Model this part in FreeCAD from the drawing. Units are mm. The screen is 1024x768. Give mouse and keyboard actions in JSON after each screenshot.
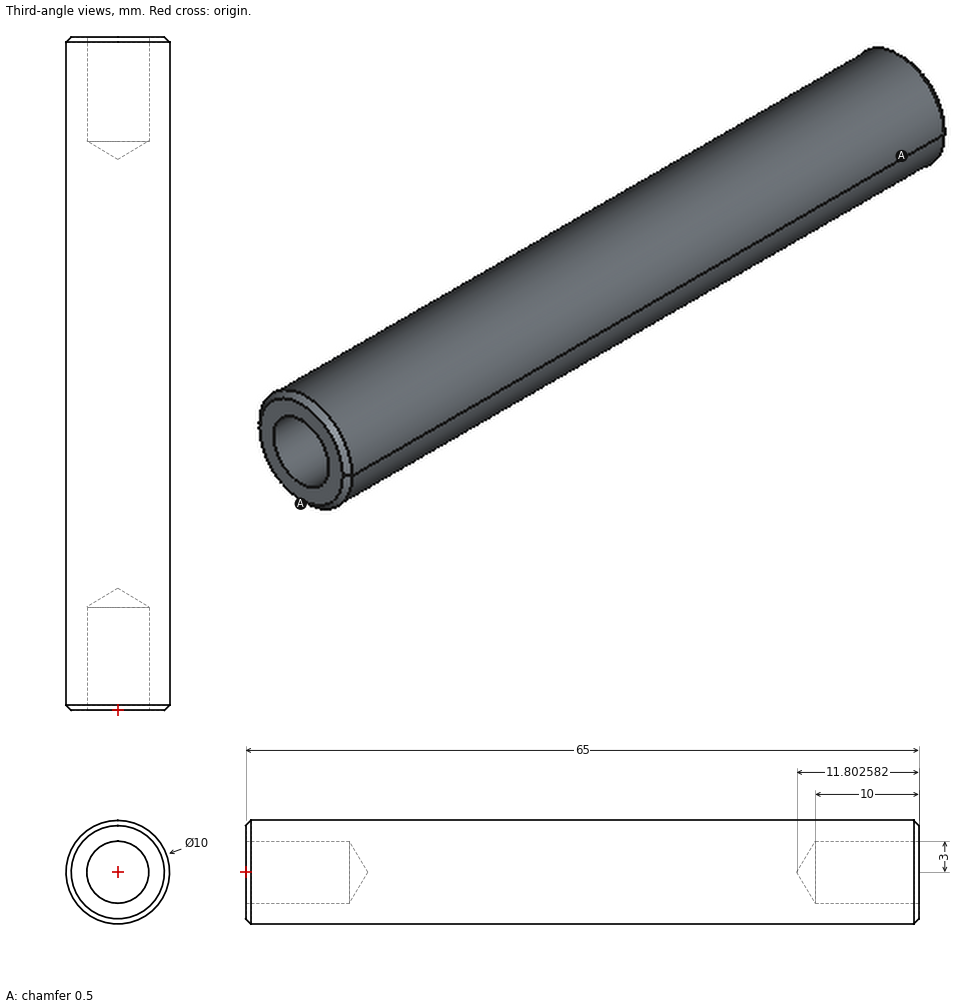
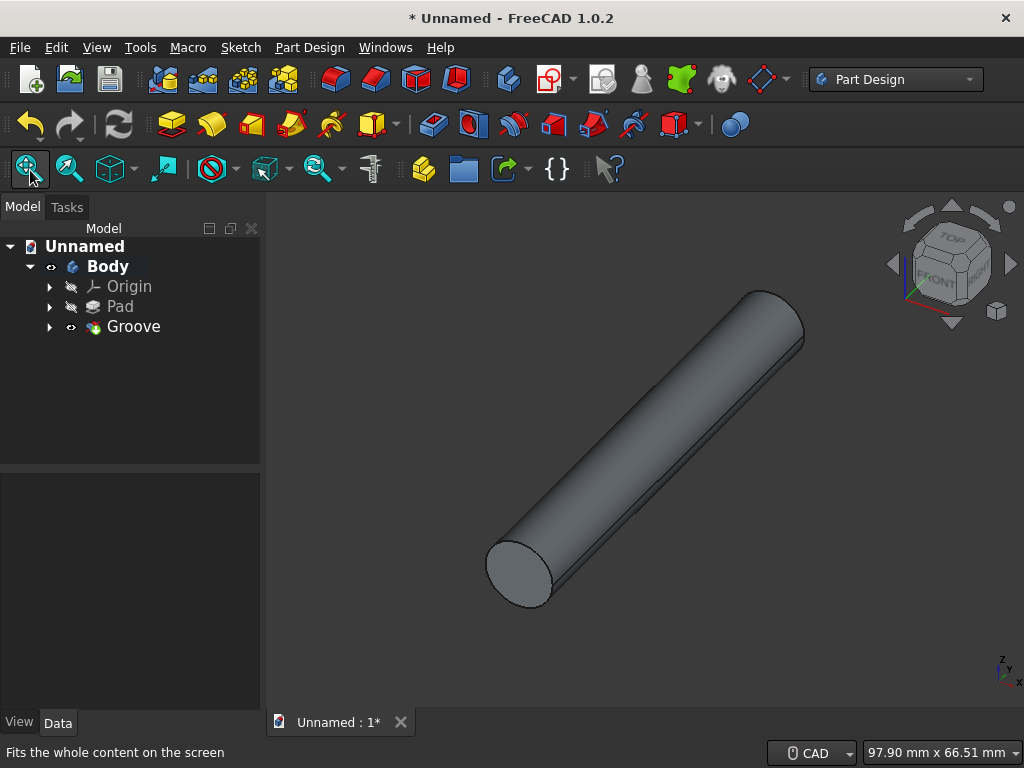
{"action": "left_click", "coordinate": [50, 287]}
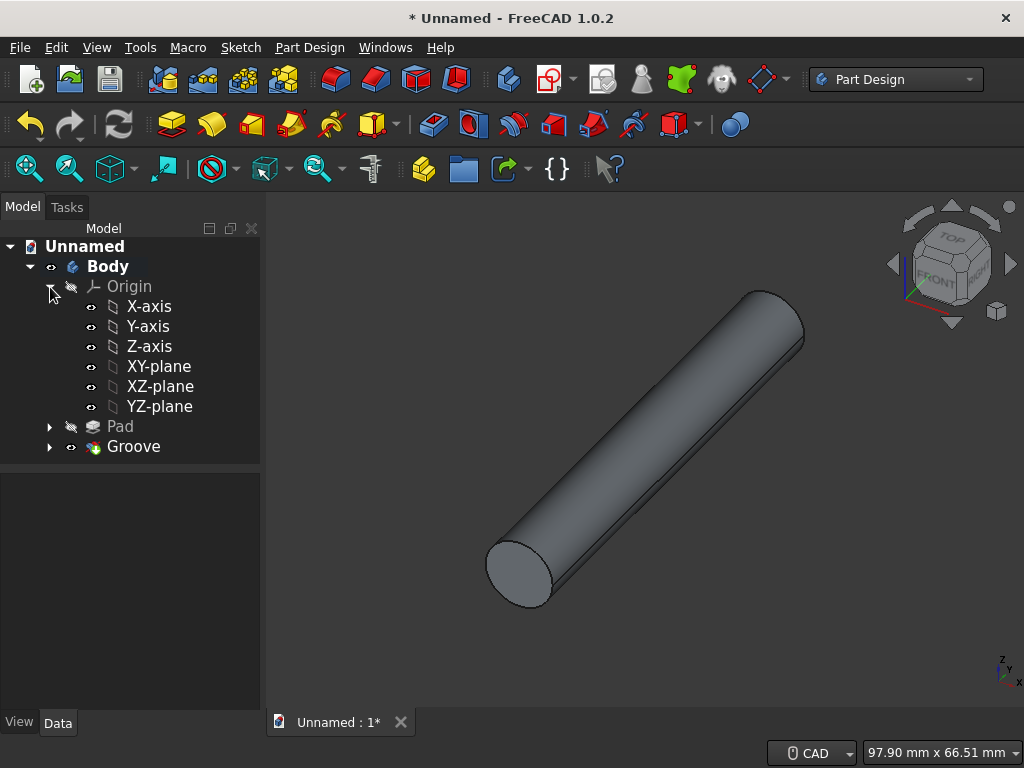
{"action": "left_click", "coordinate": [136, 387]}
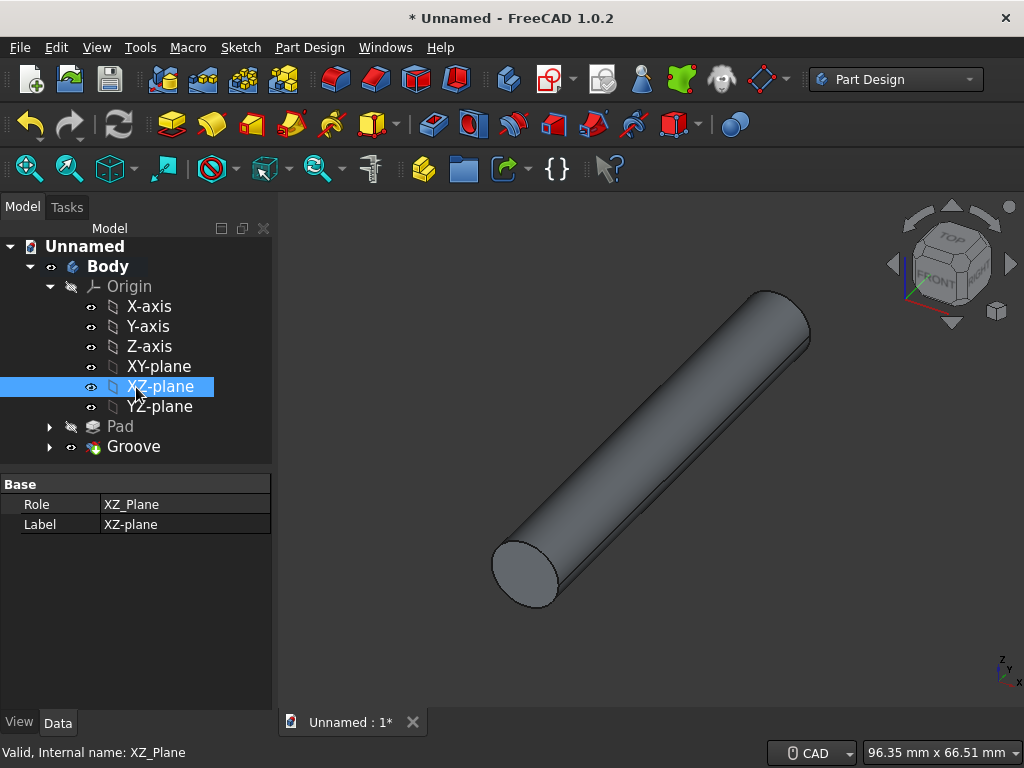
{"action": "left_click", "coordinate": [762, 80]}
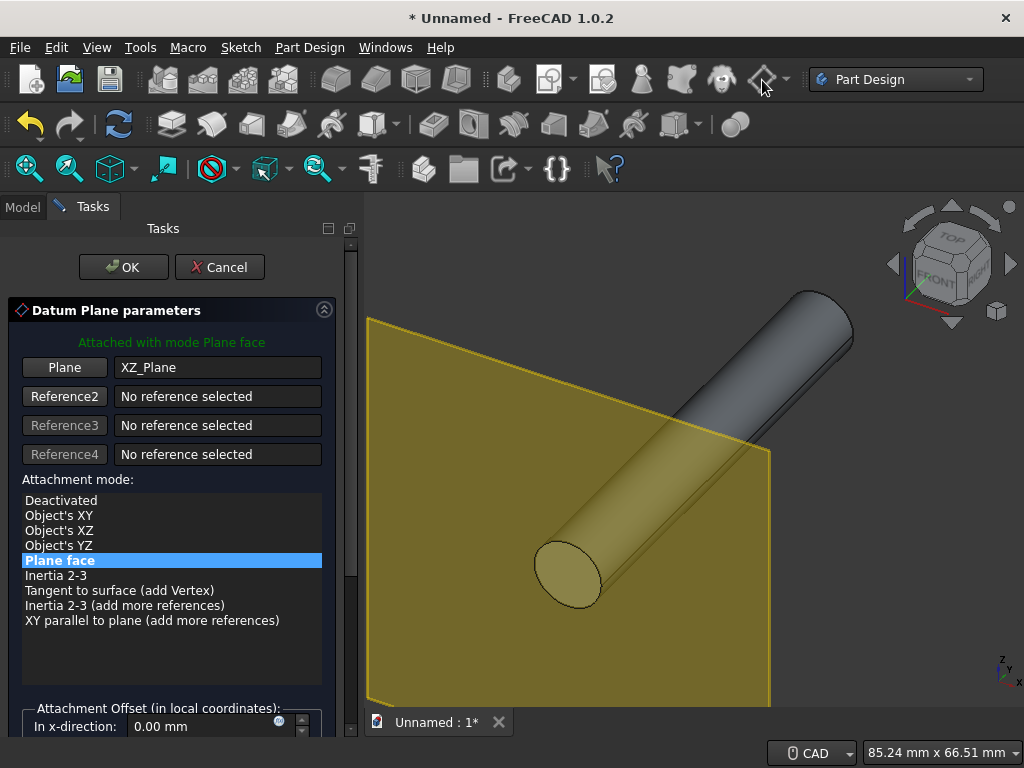
{"action": "scroll", "coordinate": [351, 487], "scroll_direction": "down", "scroll_amount": 3}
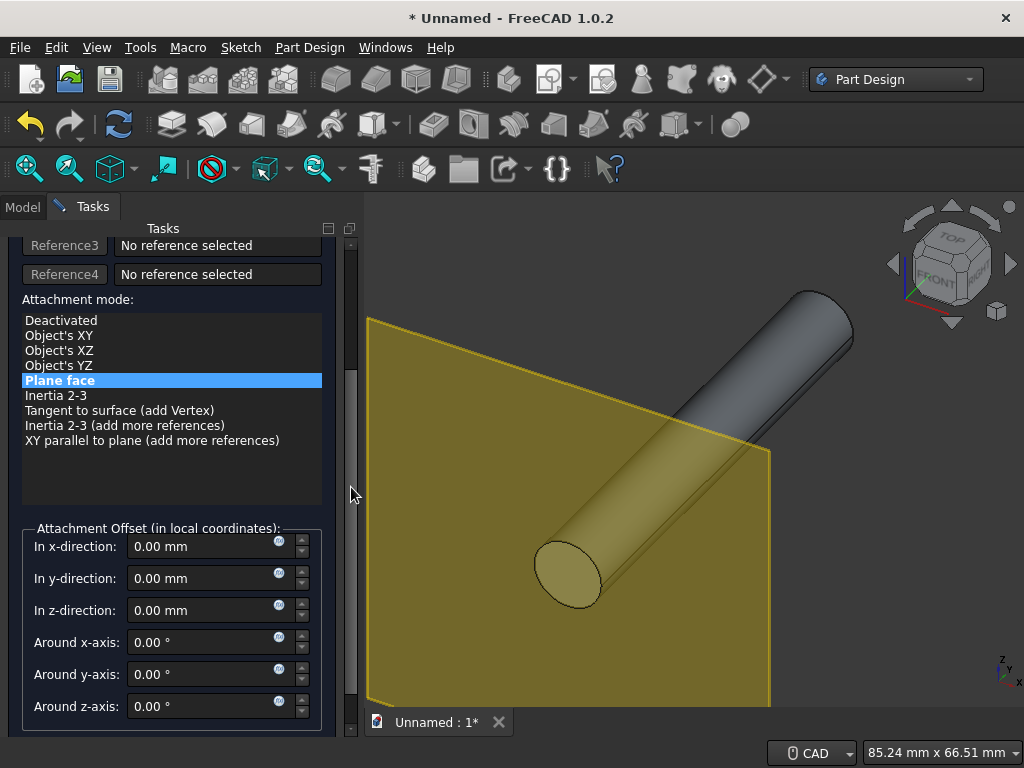
{"action": "triple_click", "coordinate": [210, 610]}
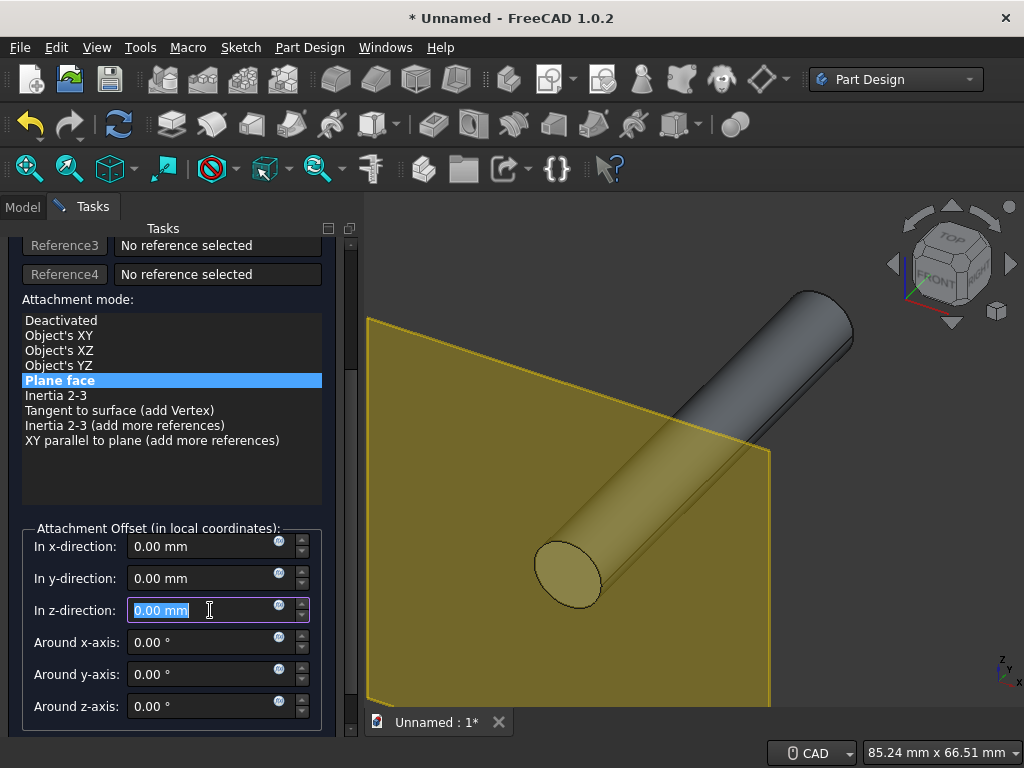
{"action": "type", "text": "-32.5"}
{"action": "key", "text": "Tab"}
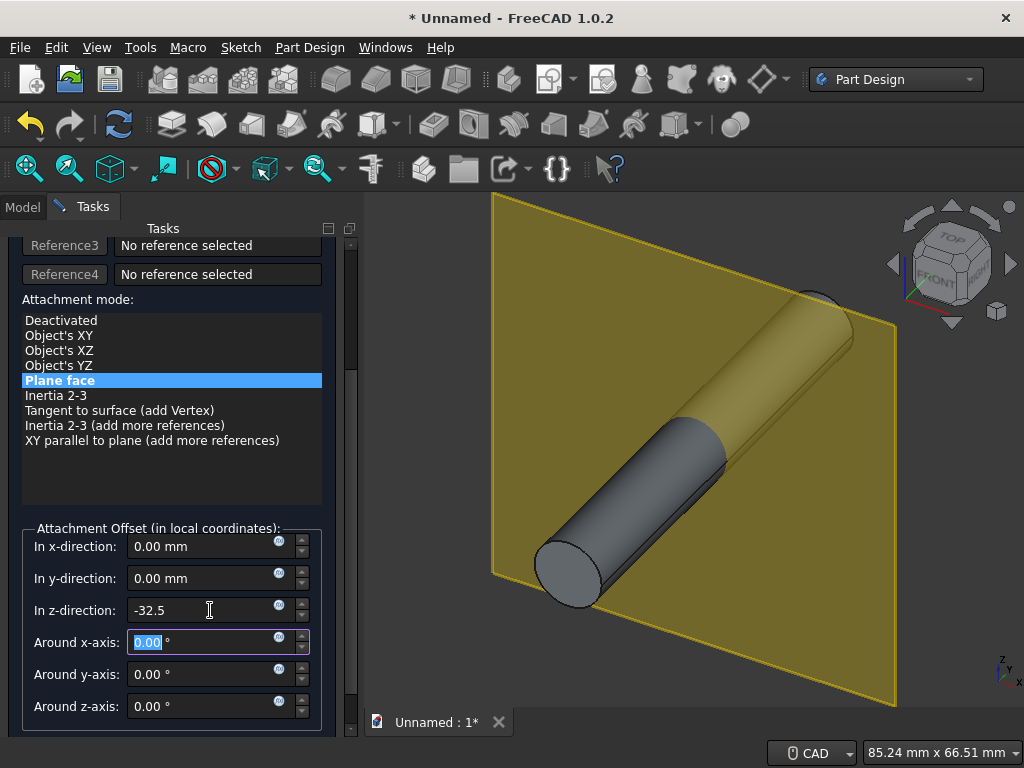
{"action": "scroll", "coordinate": [351, 487], "scroll_direction": "up", "scroll_amount": 4}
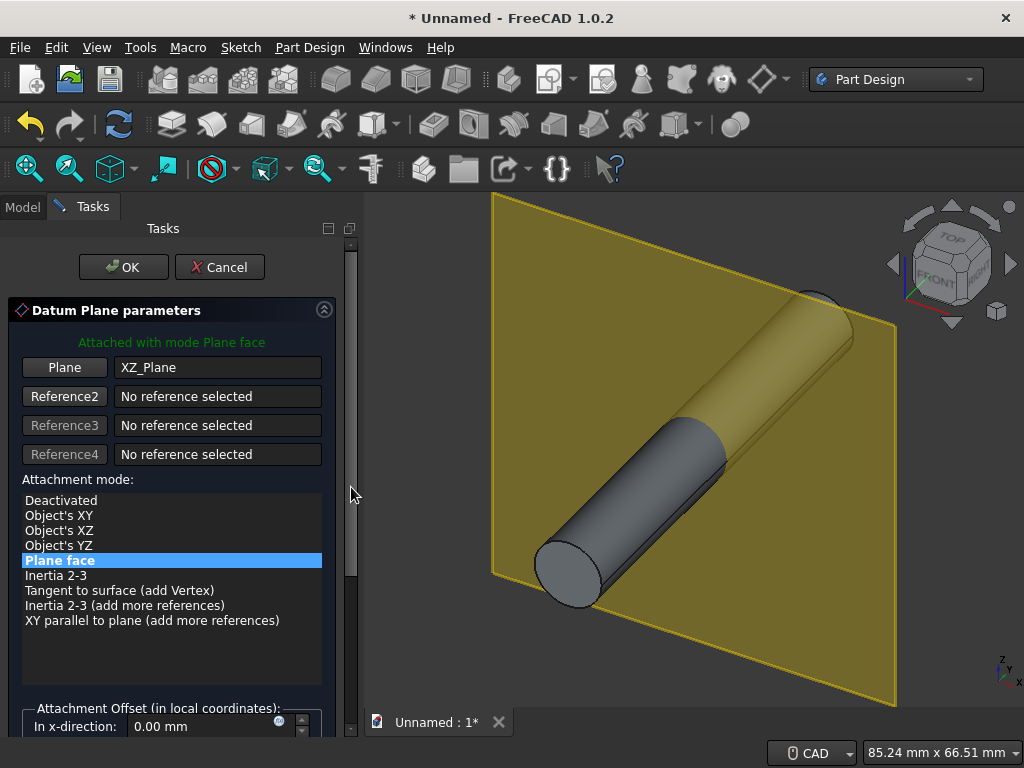
{"action": "left_click", "coordinate": [124, 267]}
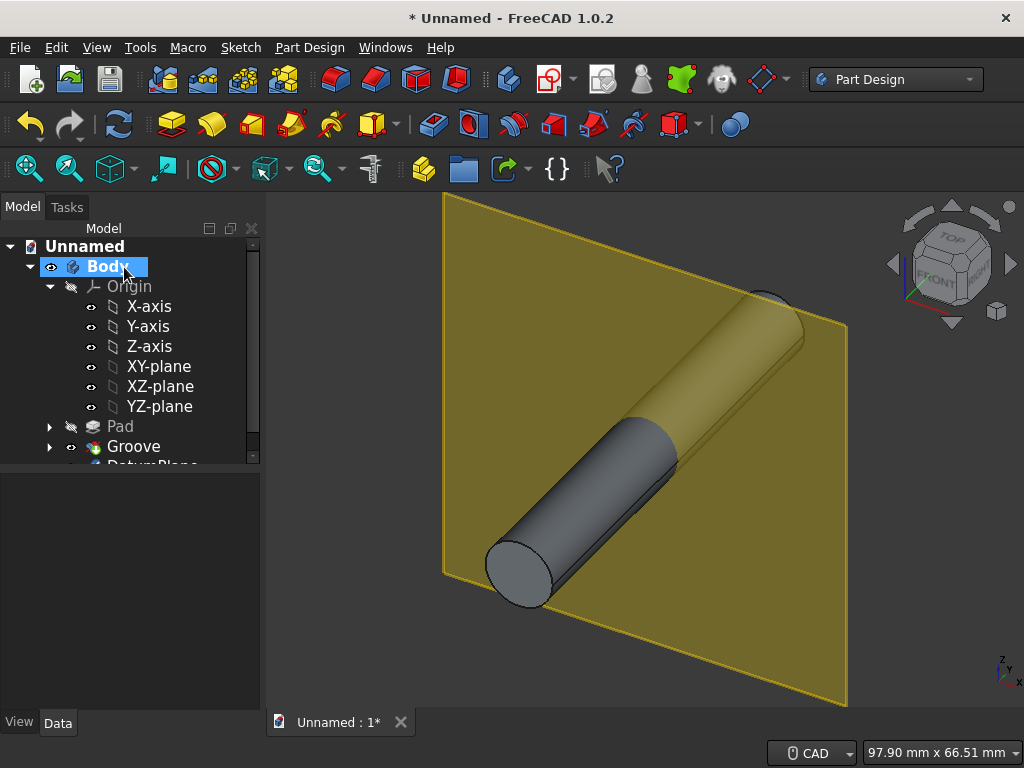
{"action": "left_click", "coordinate": [116, 447]}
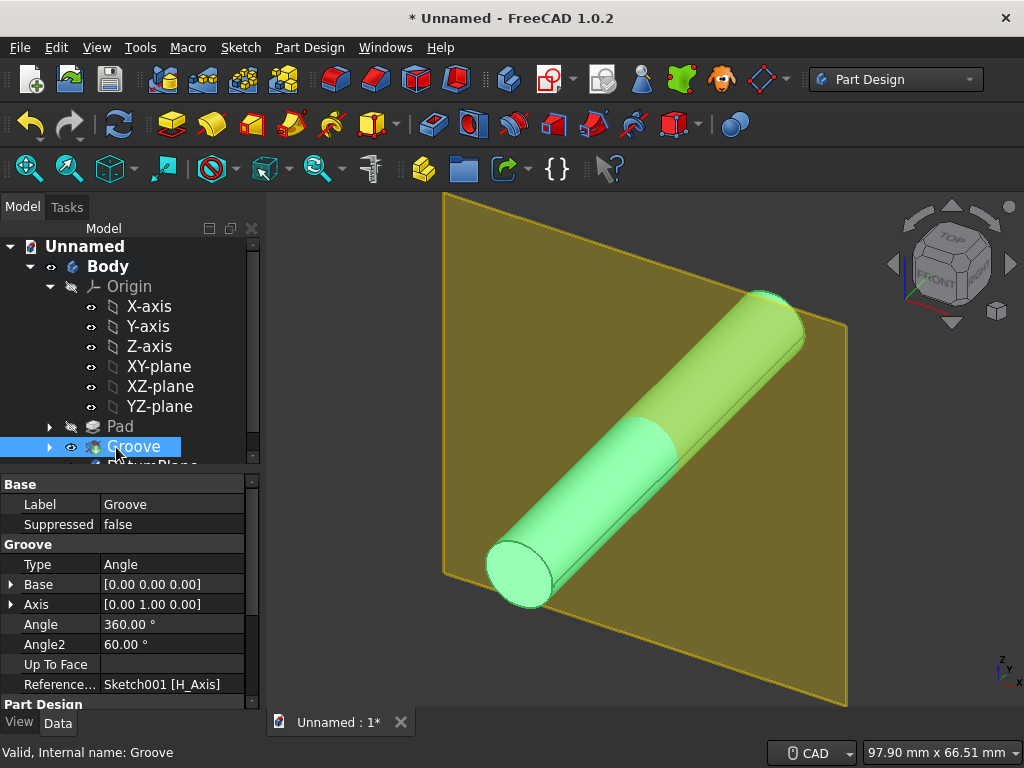
{"action": "left_click", "coordinate": [164, 80]}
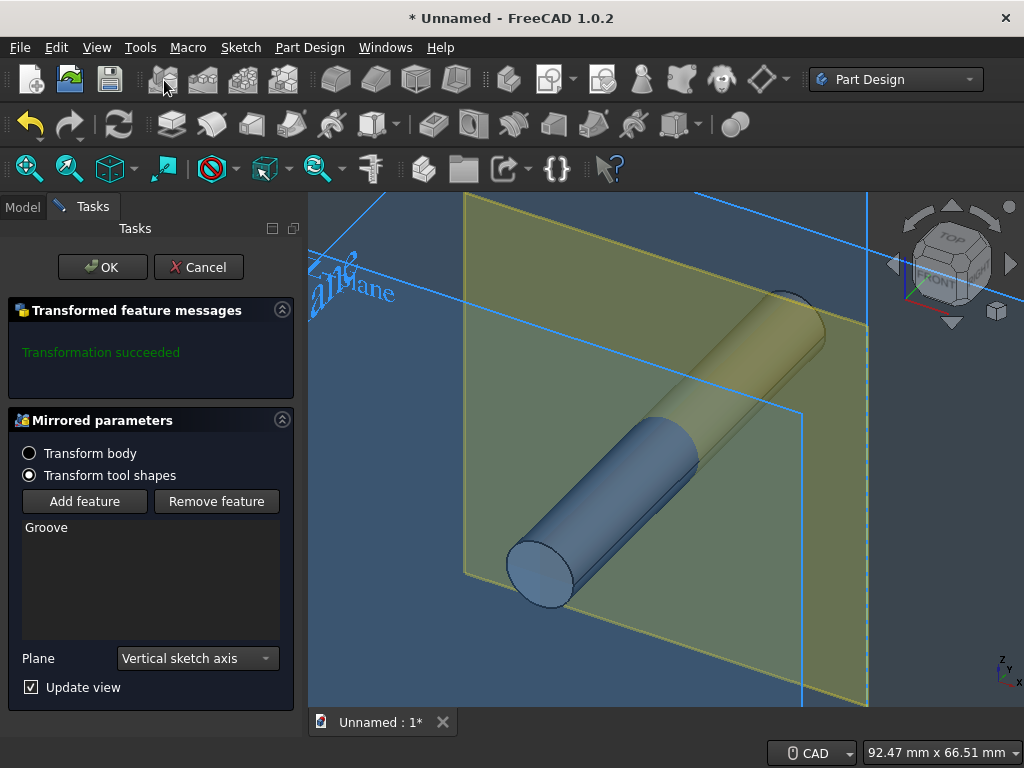
{"action": "left_click", "coordinate": [198, 658]}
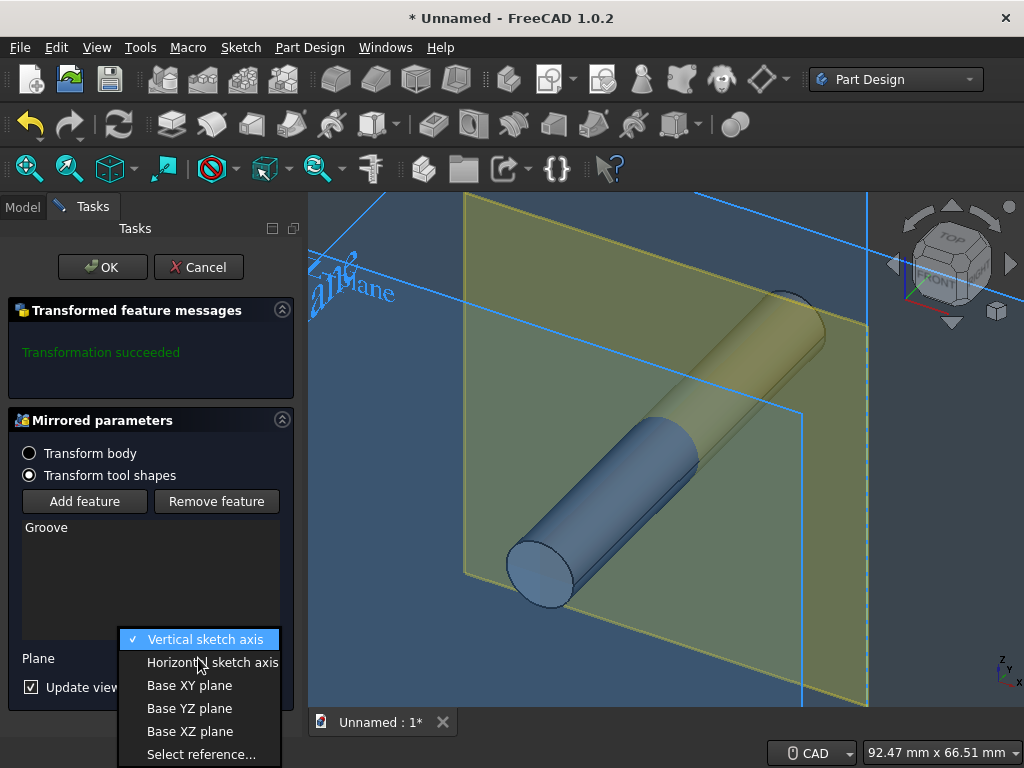
{"action": "left_click", "coordinate": [198, 754]}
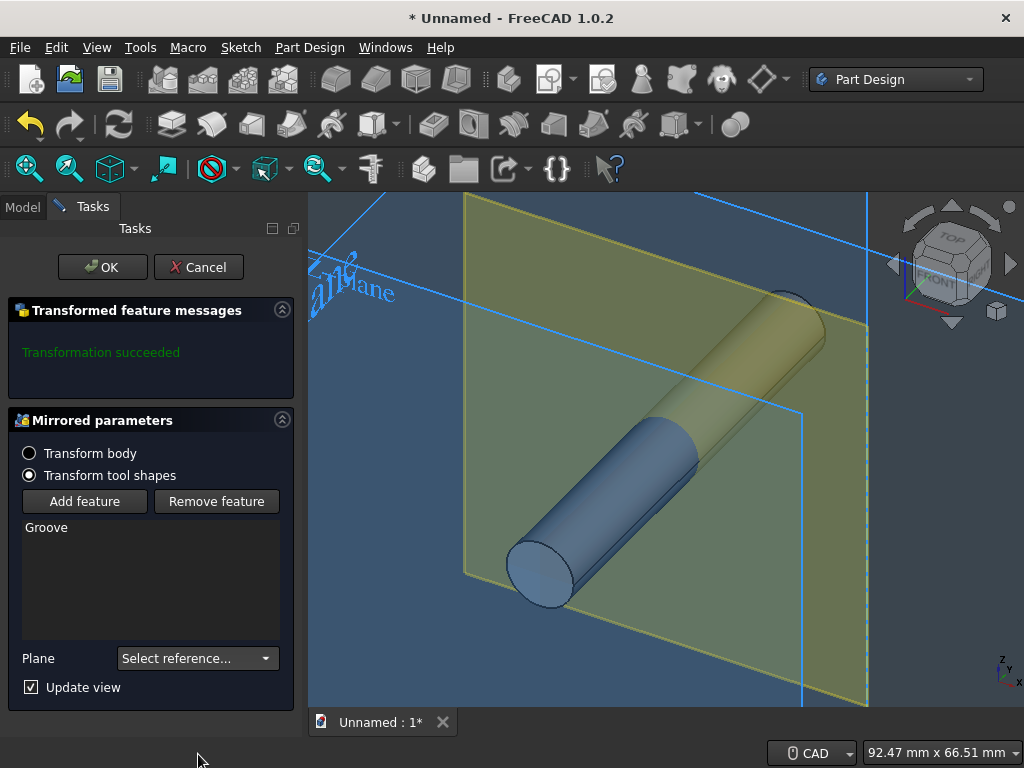
{"action": "left_click", "coordinate": [23, 206]}